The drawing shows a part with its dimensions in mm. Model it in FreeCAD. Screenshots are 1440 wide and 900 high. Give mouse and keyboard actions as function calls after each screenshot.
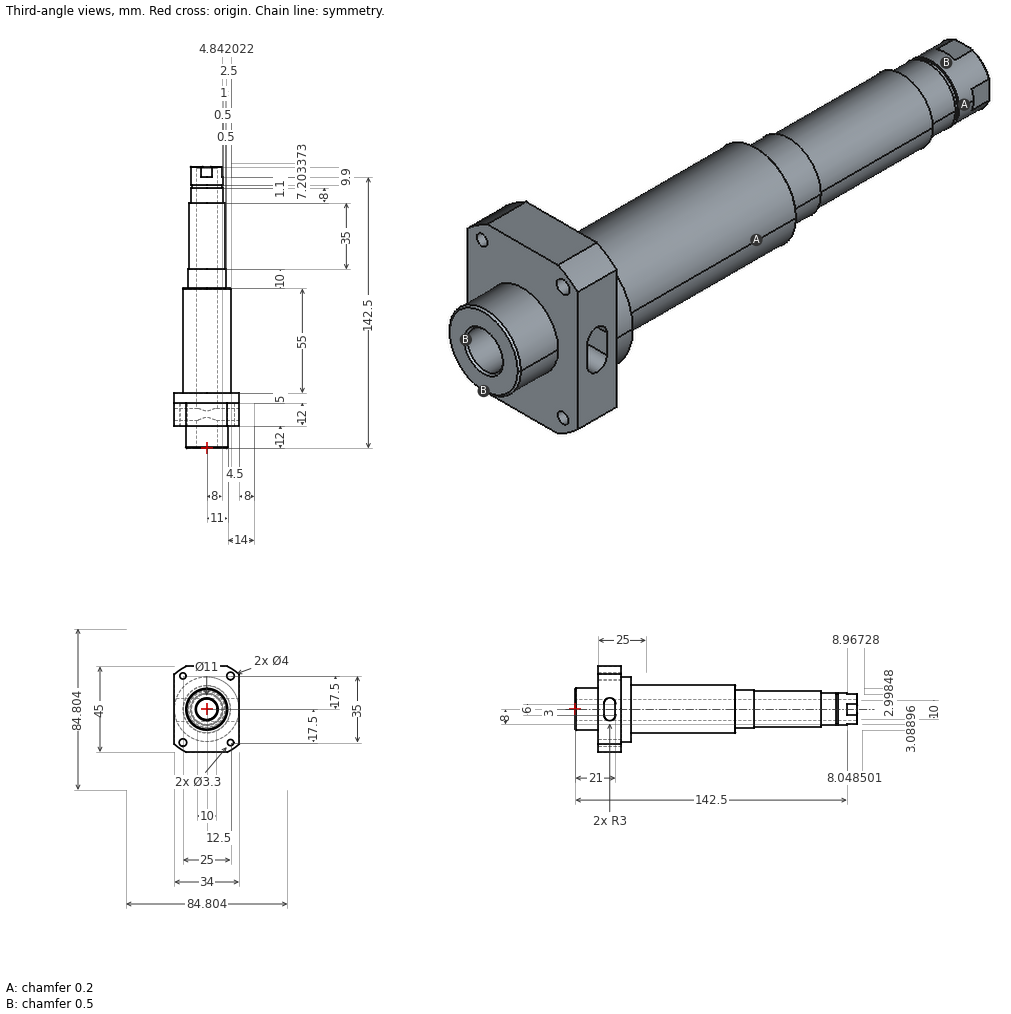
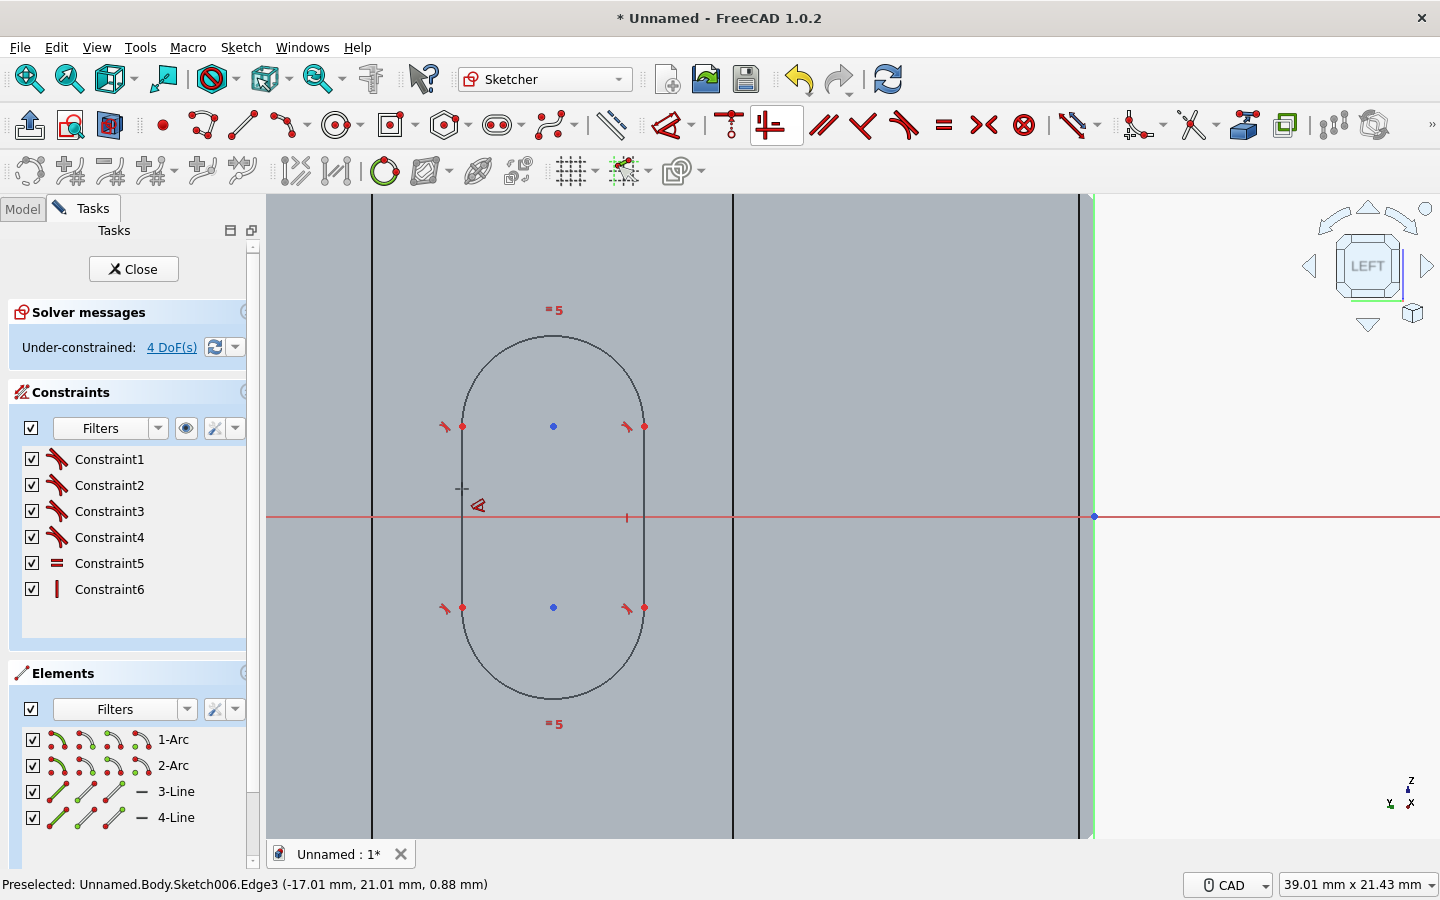
click(500, 682)
click(481, 708)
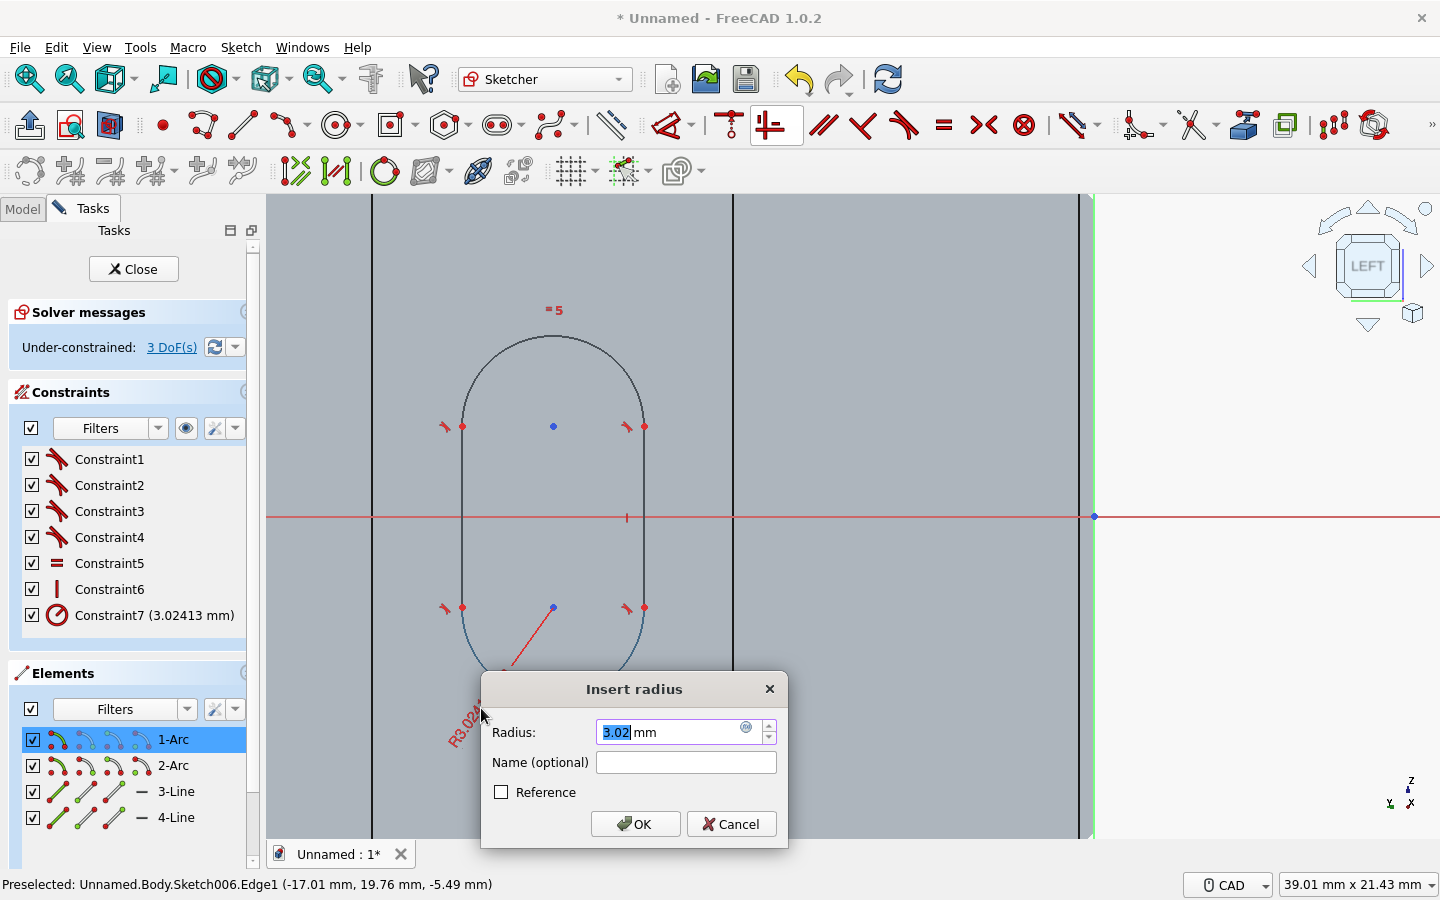
text(3)
key(Return)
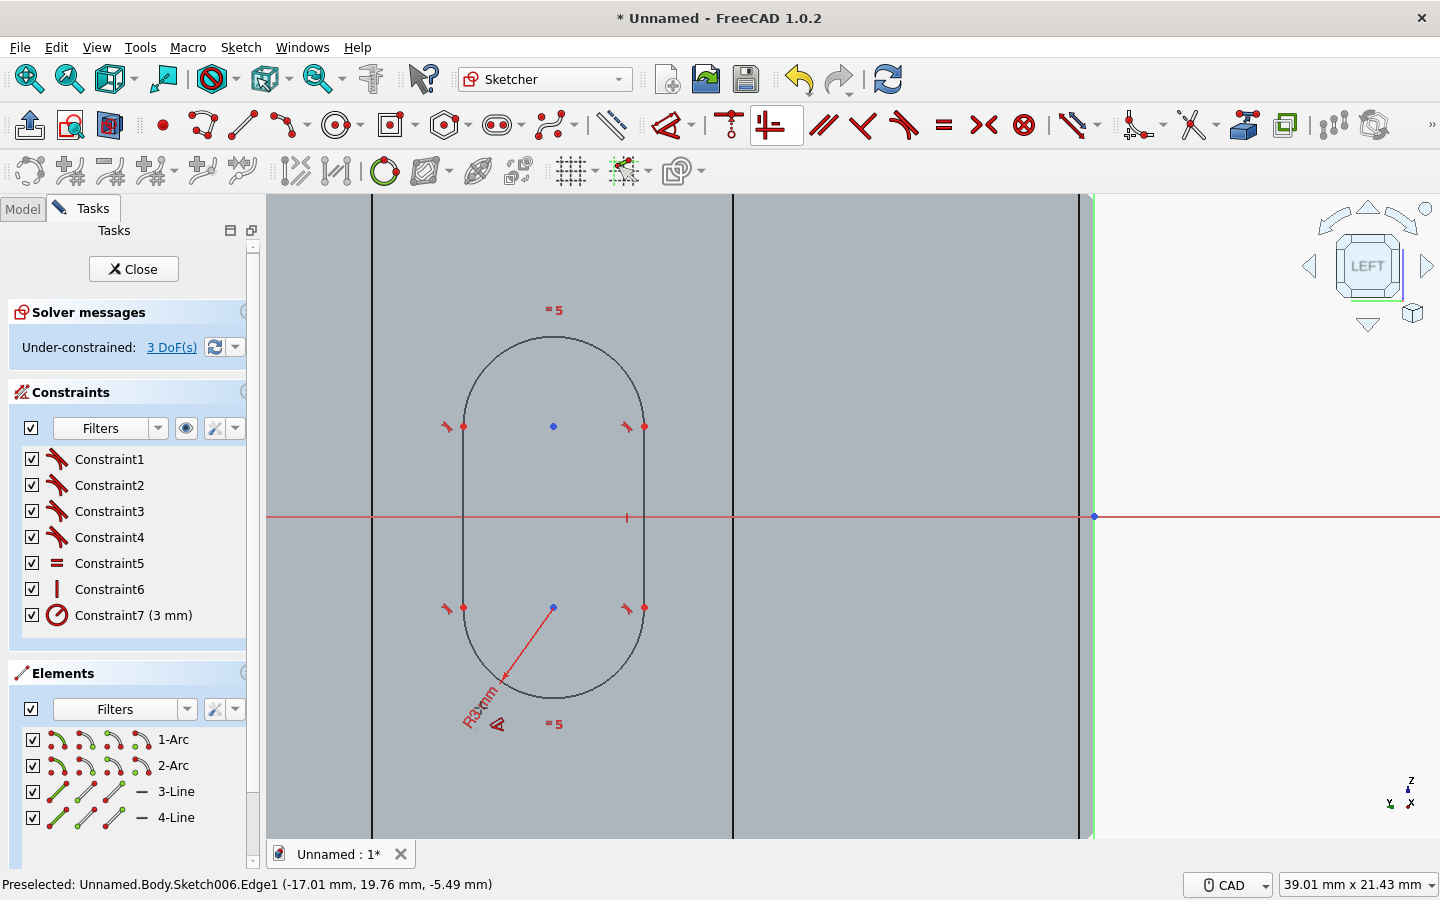
click(463, 554)
click(429, 476)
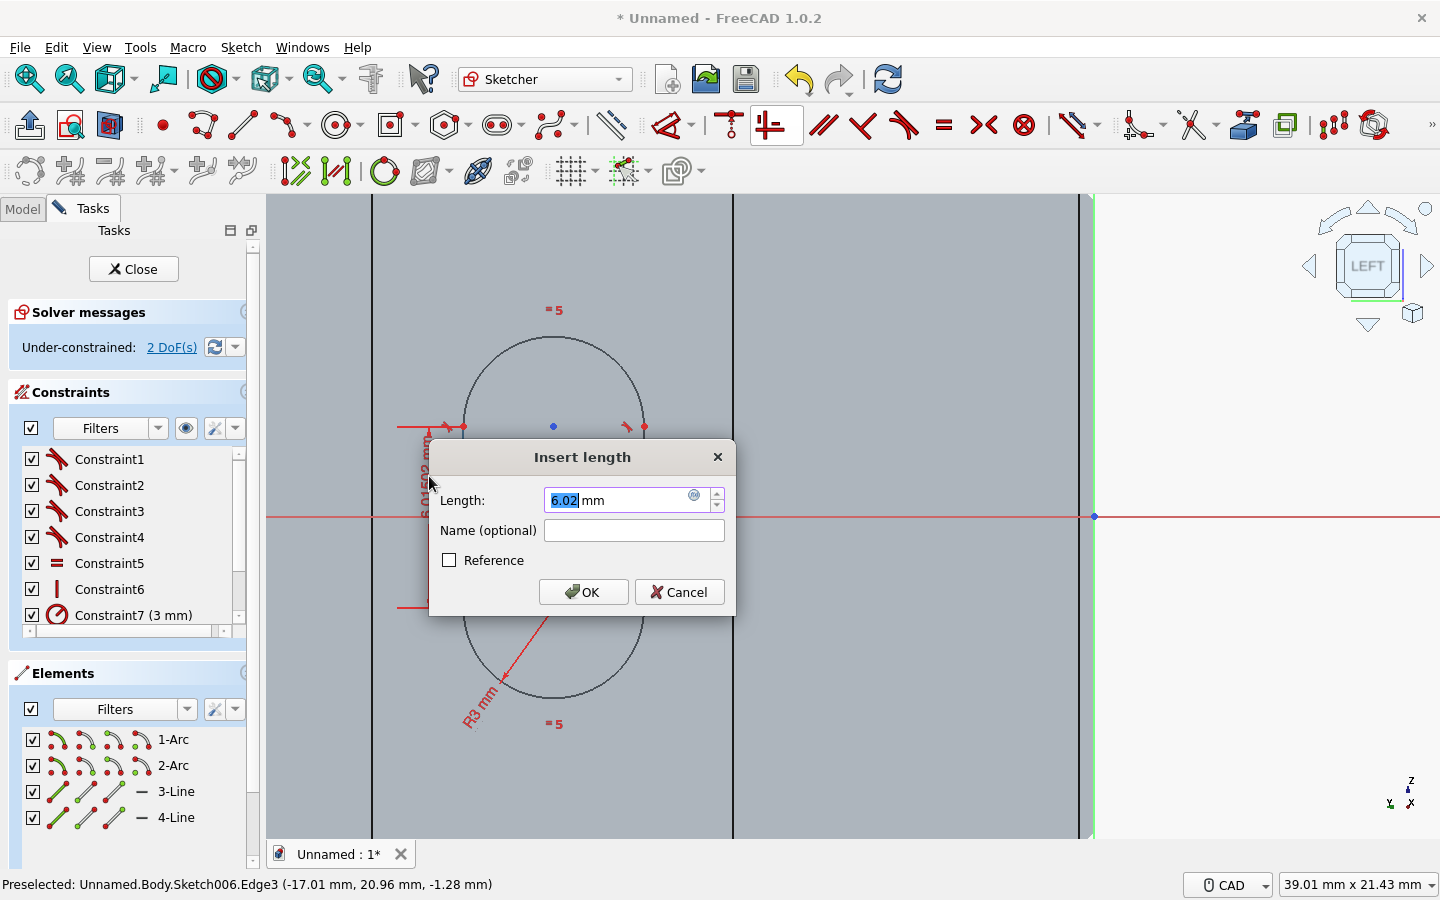
text(6)
key(Return)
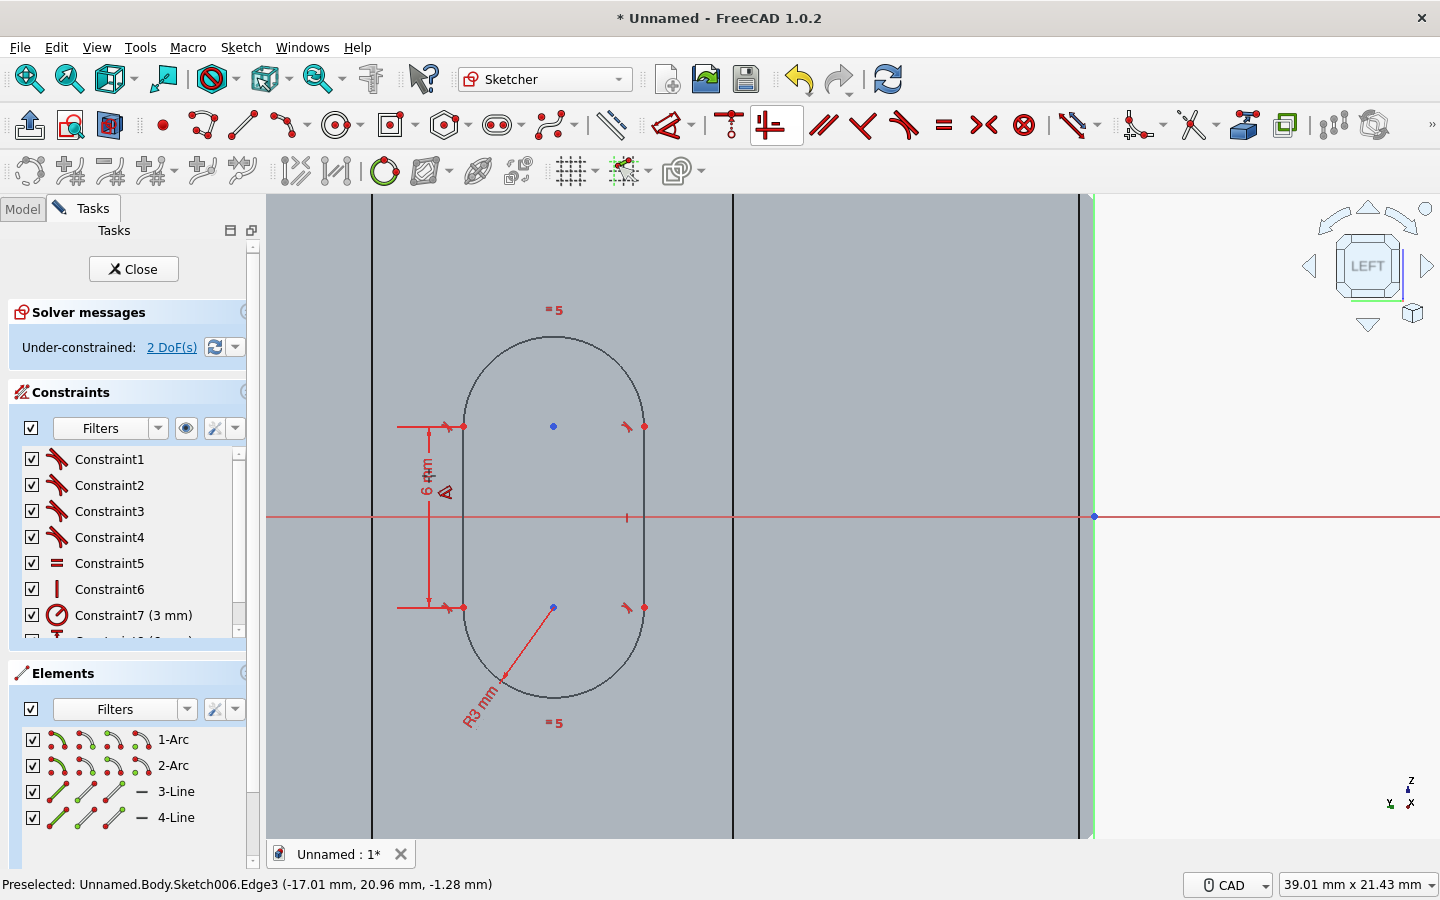
click(463, 608)
click(1128, 562)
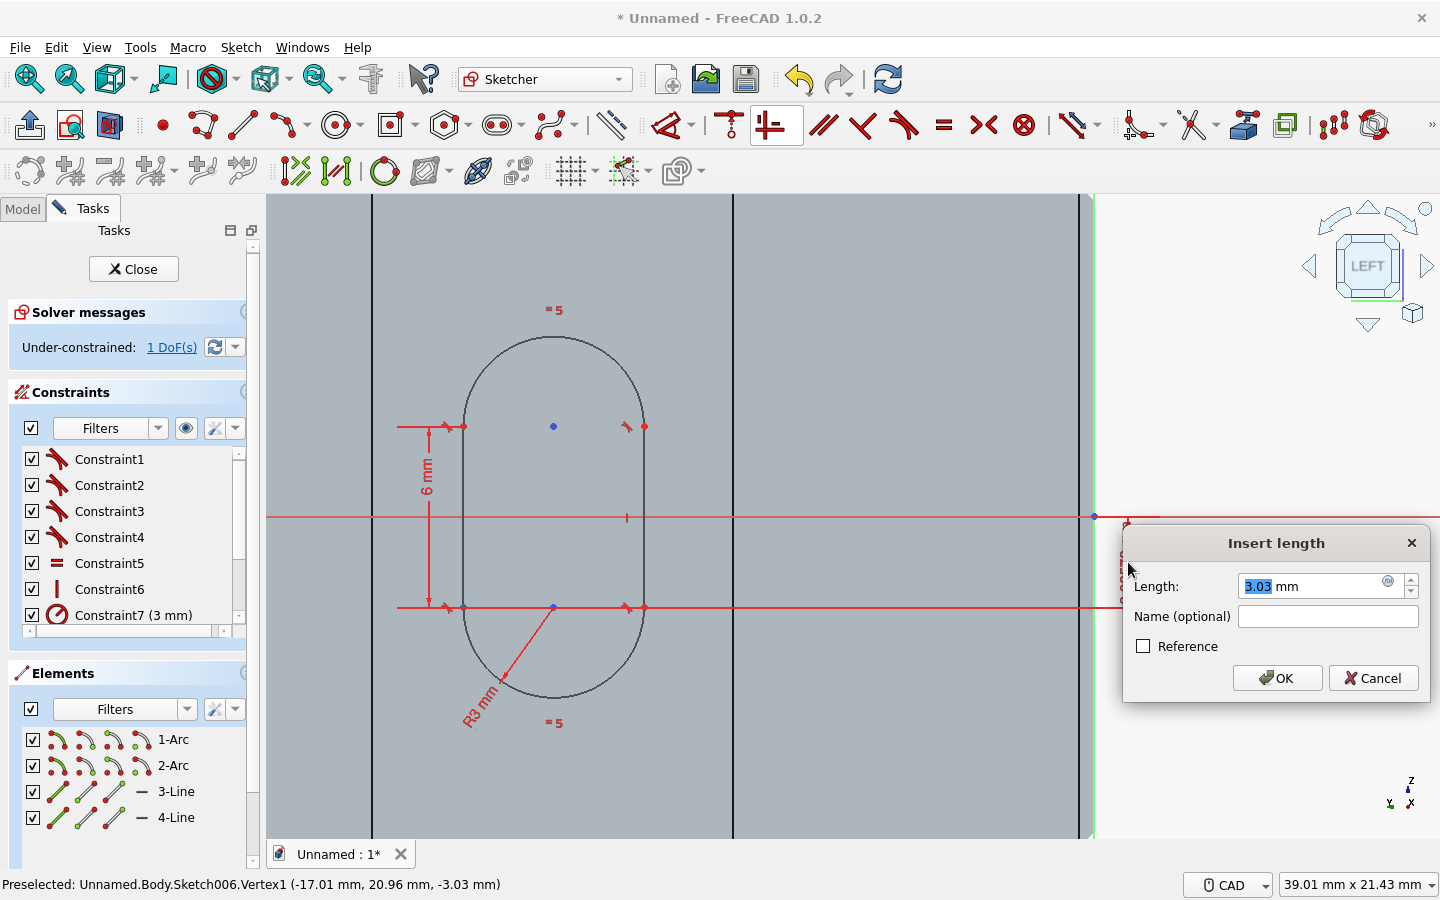
text(3)
key(Return)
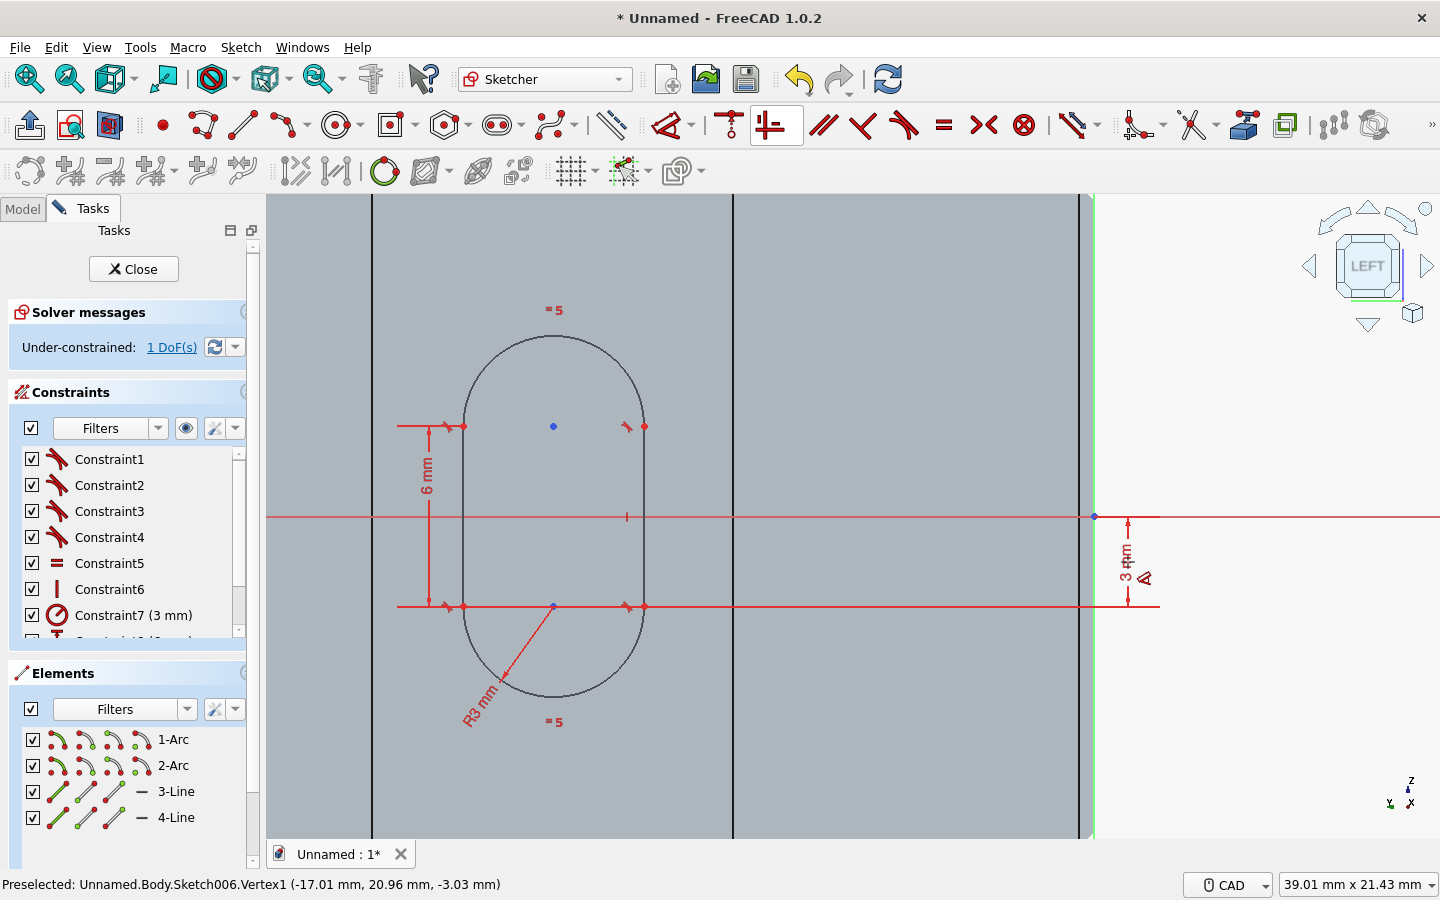
click(463, 607)
click(779, 641)